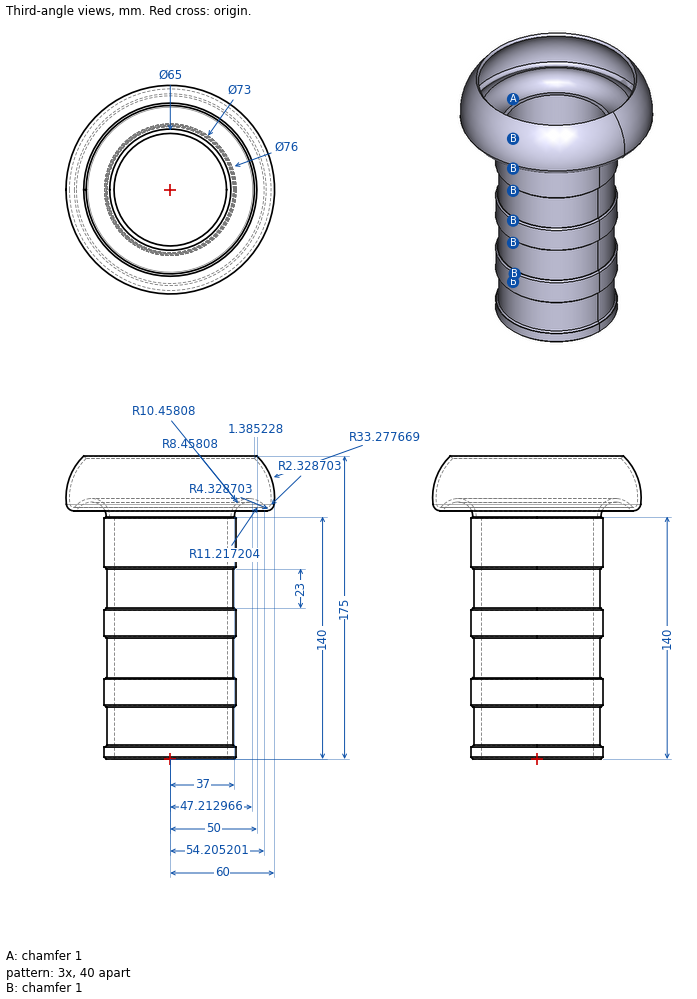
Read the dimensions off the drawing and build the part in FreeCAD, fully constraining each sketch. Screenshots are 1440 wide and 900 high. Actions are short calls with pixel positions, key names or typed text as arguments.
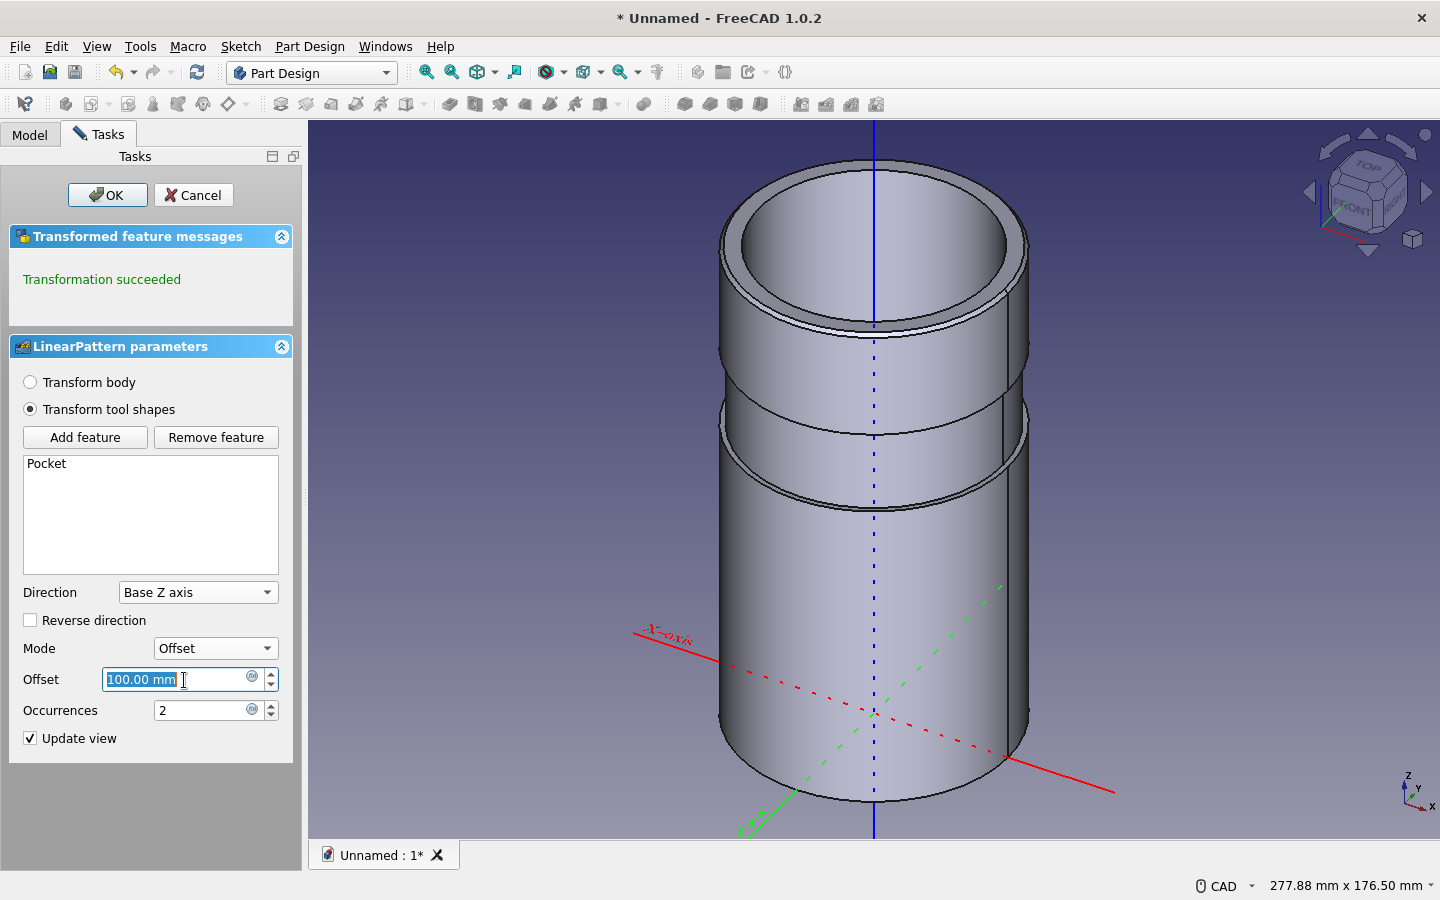
text(40)
key(Tab)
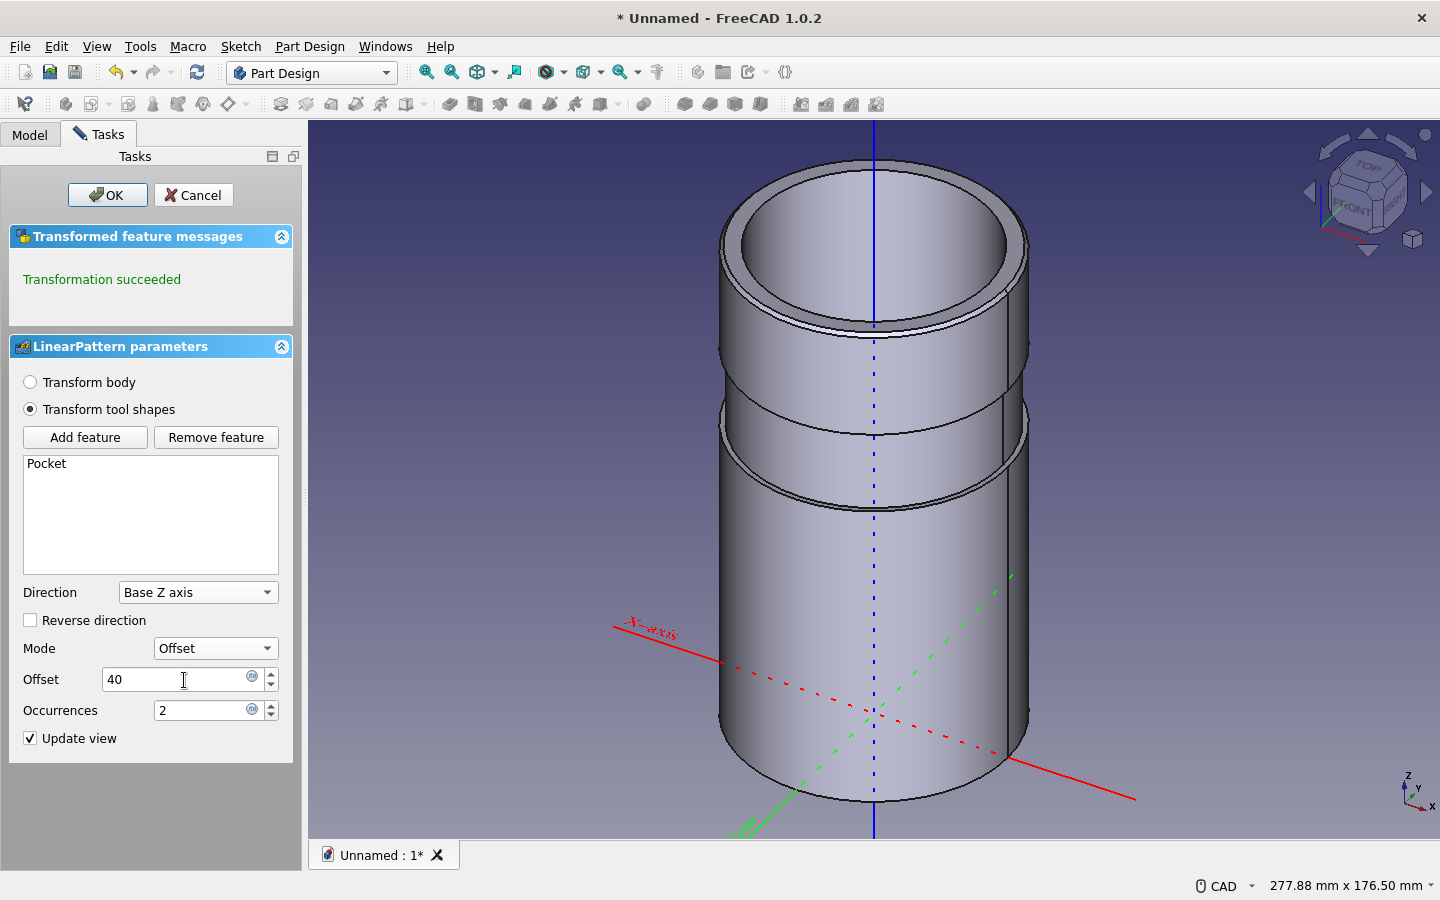
triple_click(210, 710)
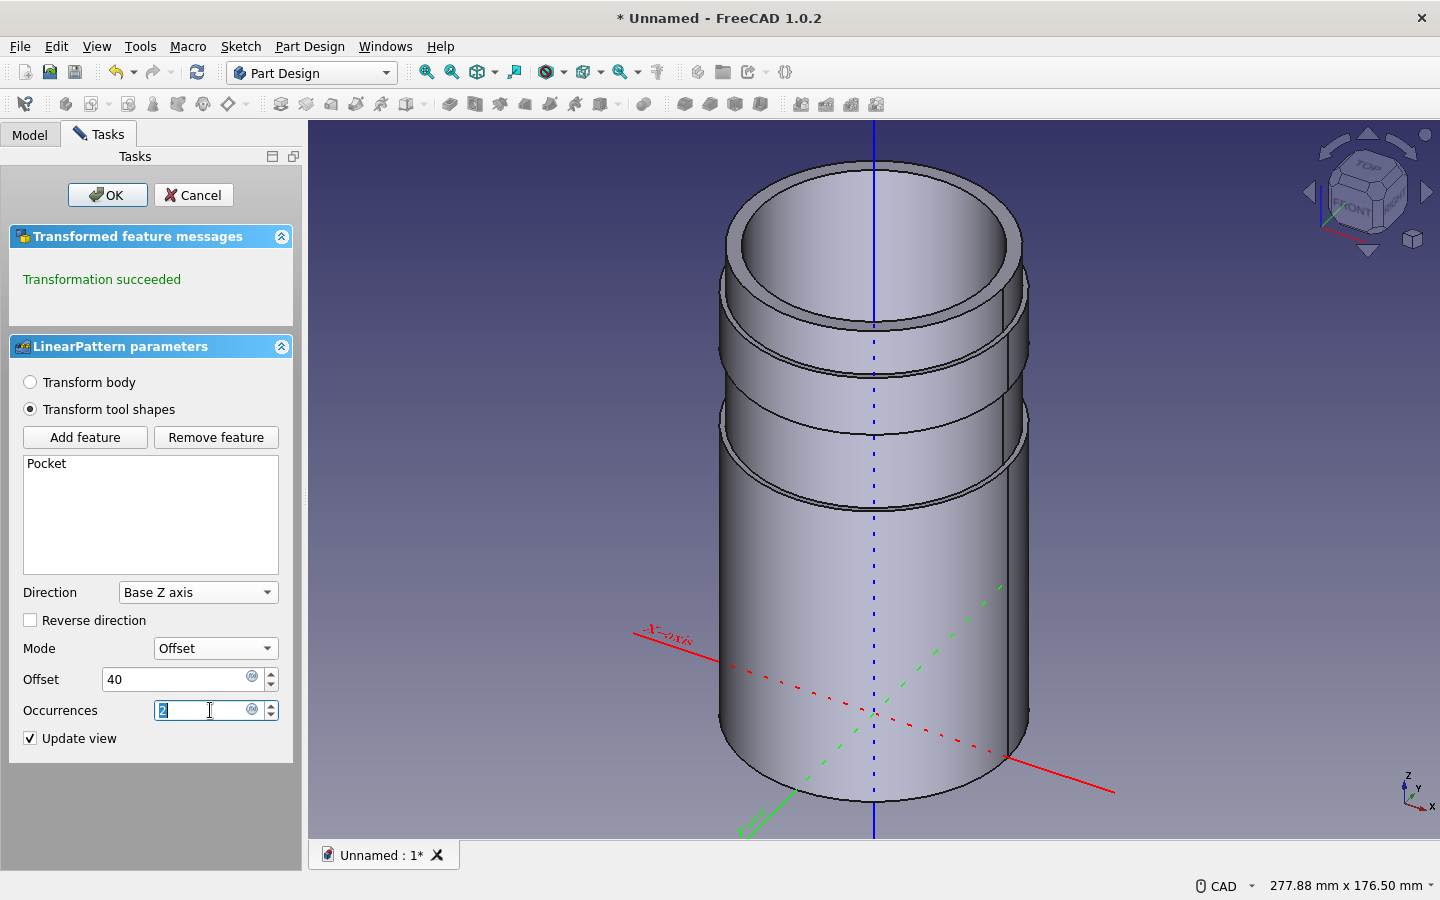
text(3)
key(Tab)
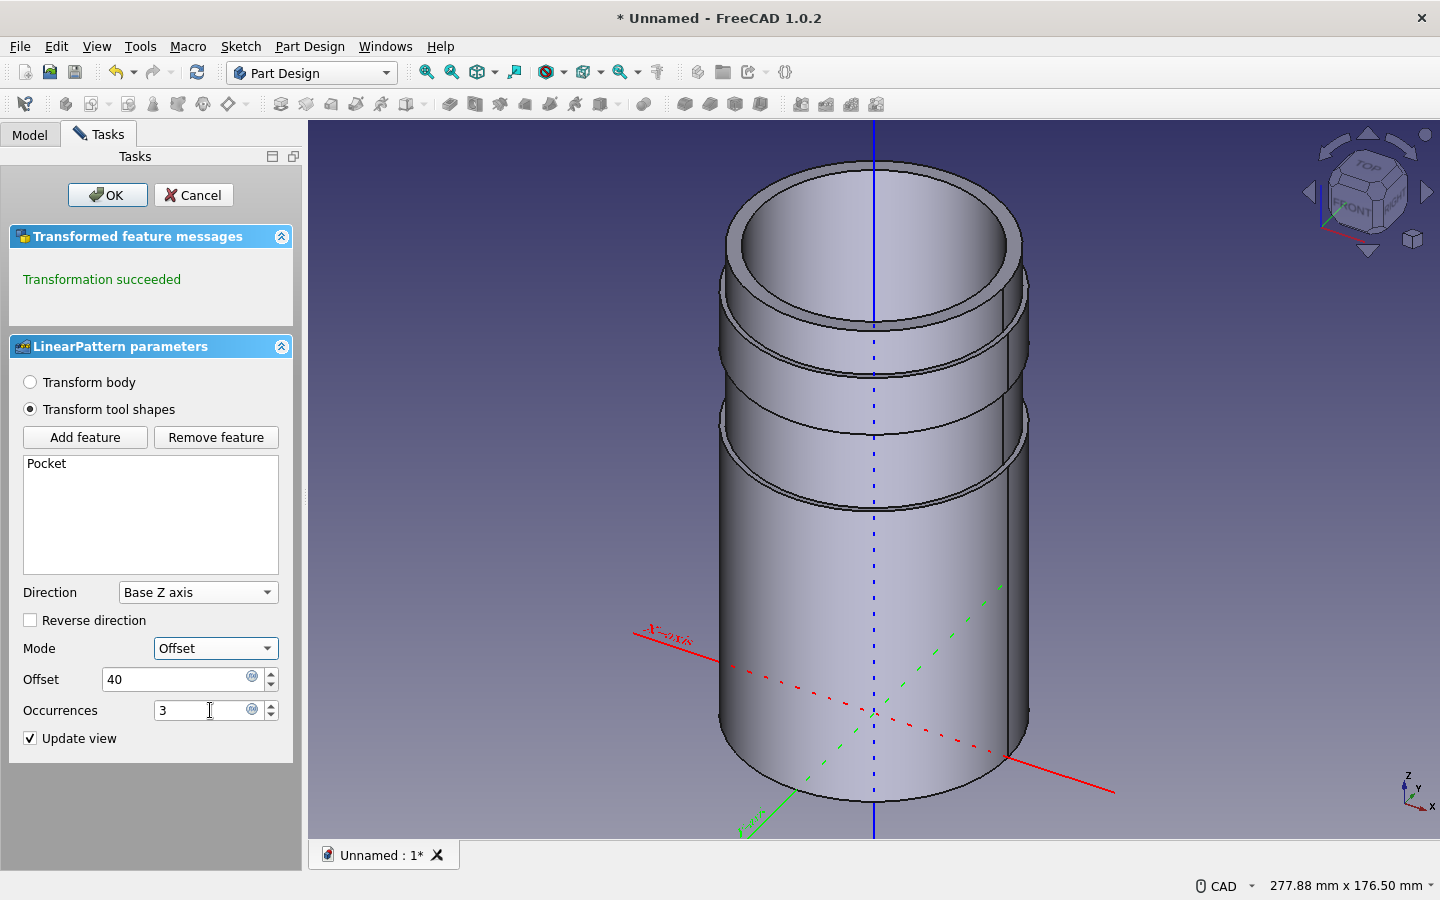
click(31, 620)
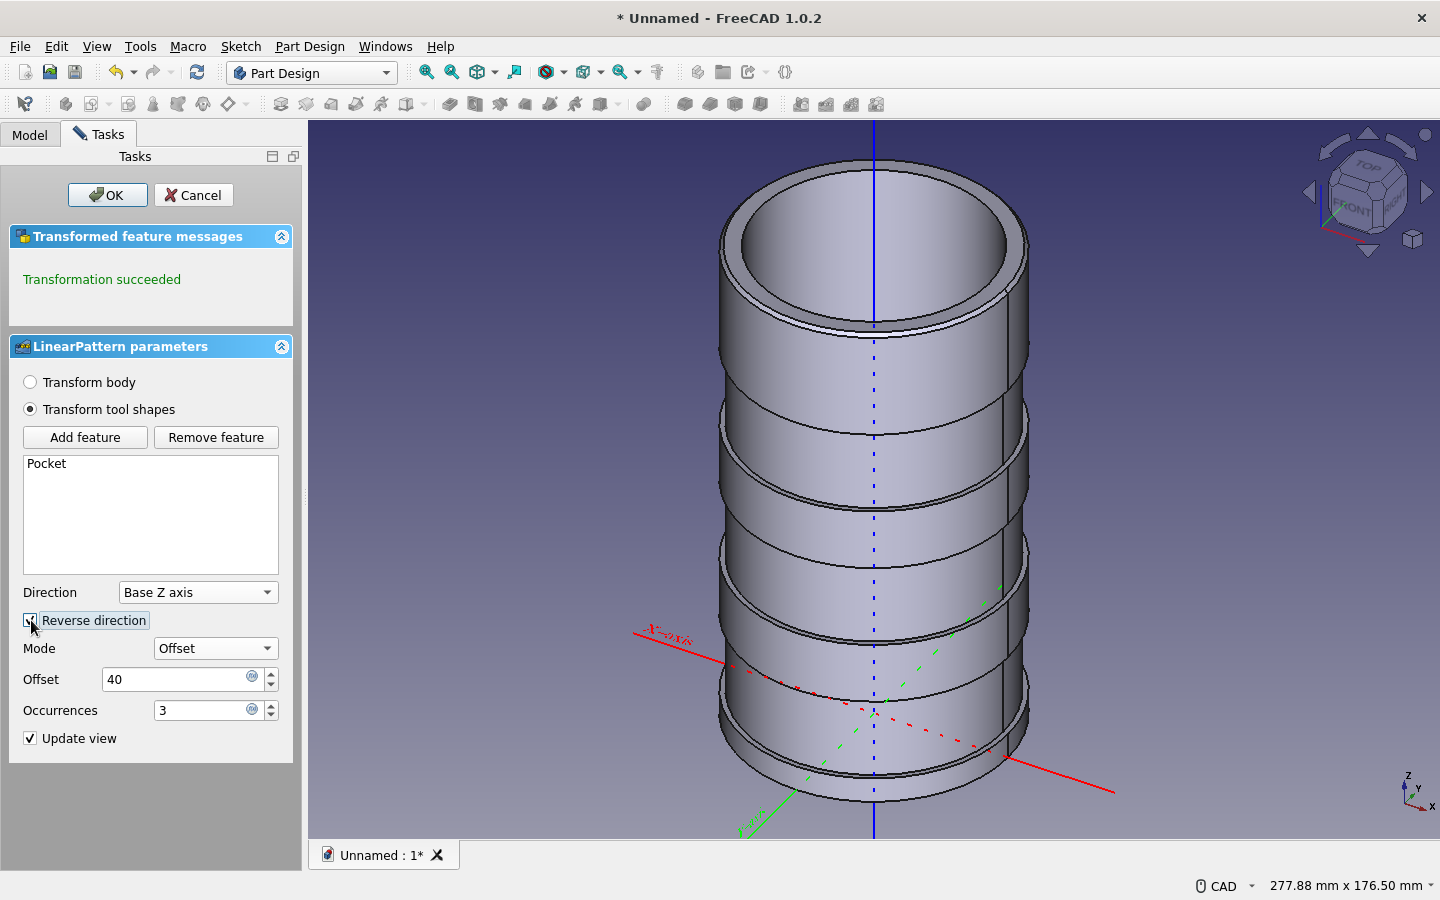
click(108, 195)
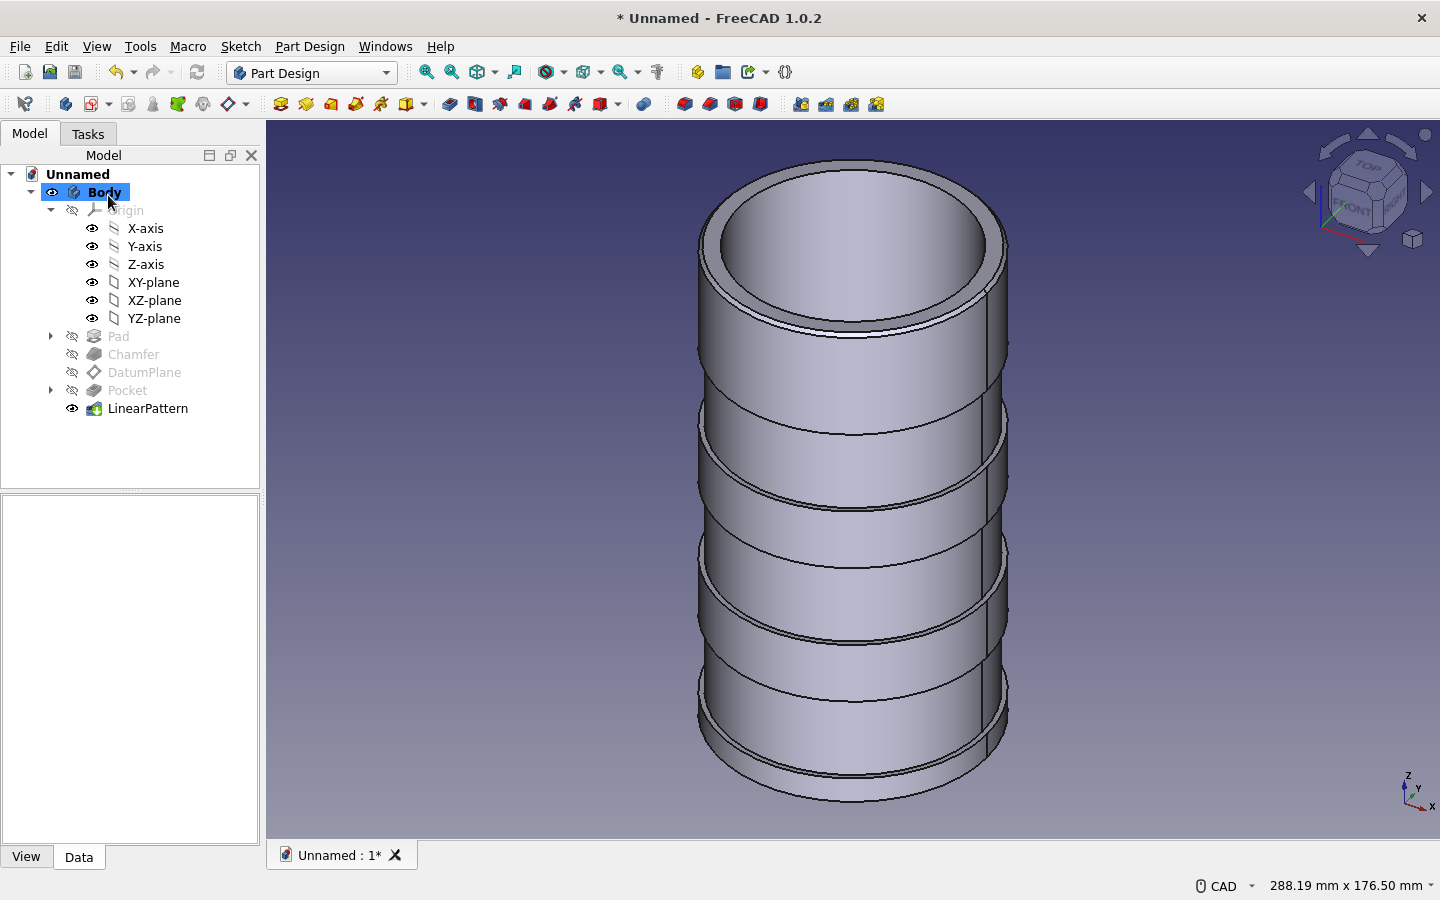
click(699, 431)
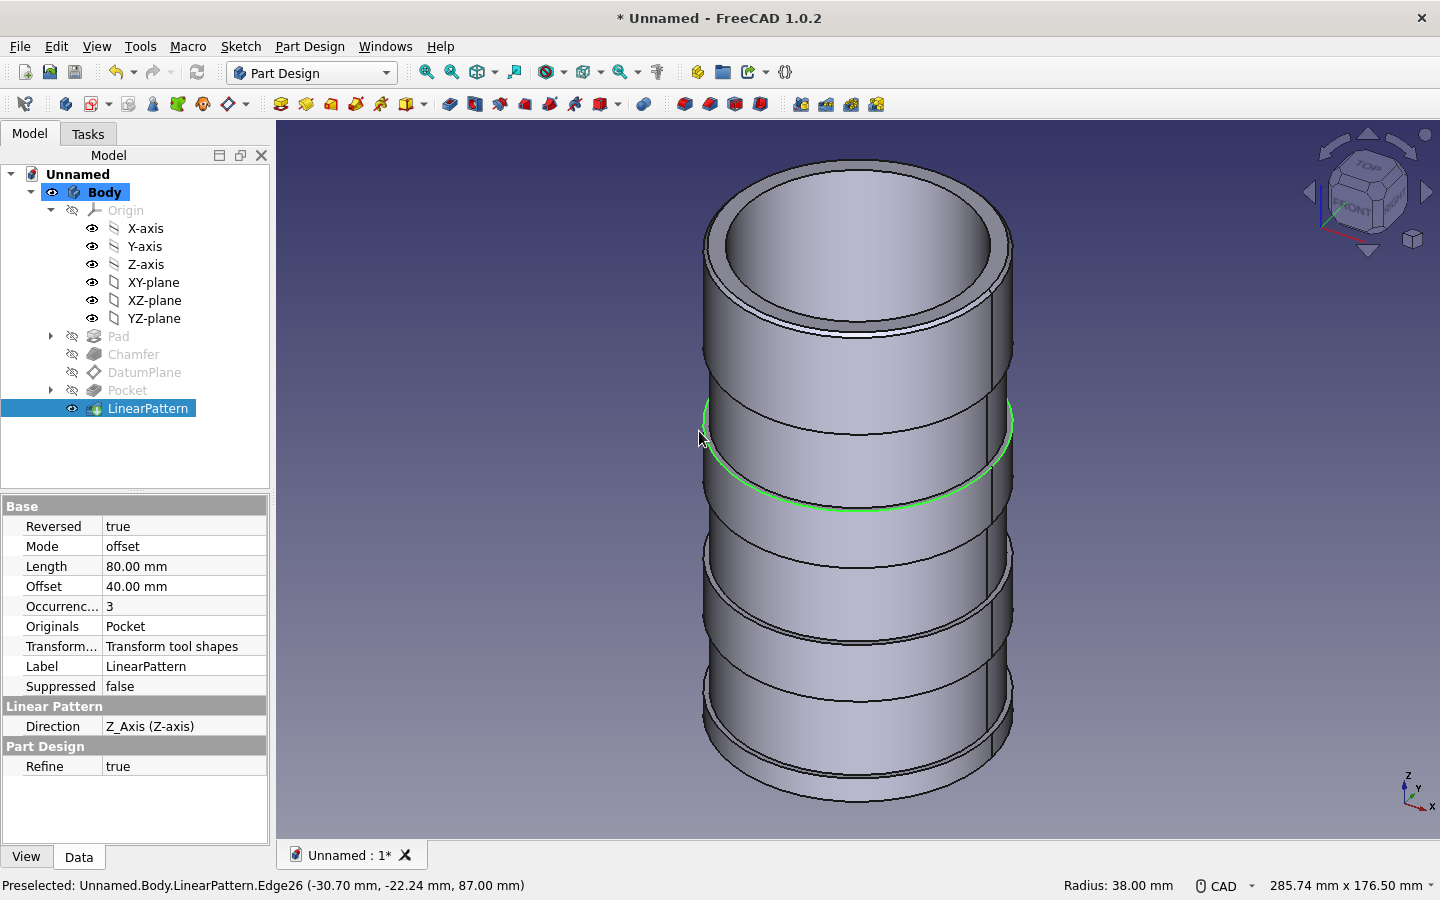
click(704, 565, ctrl)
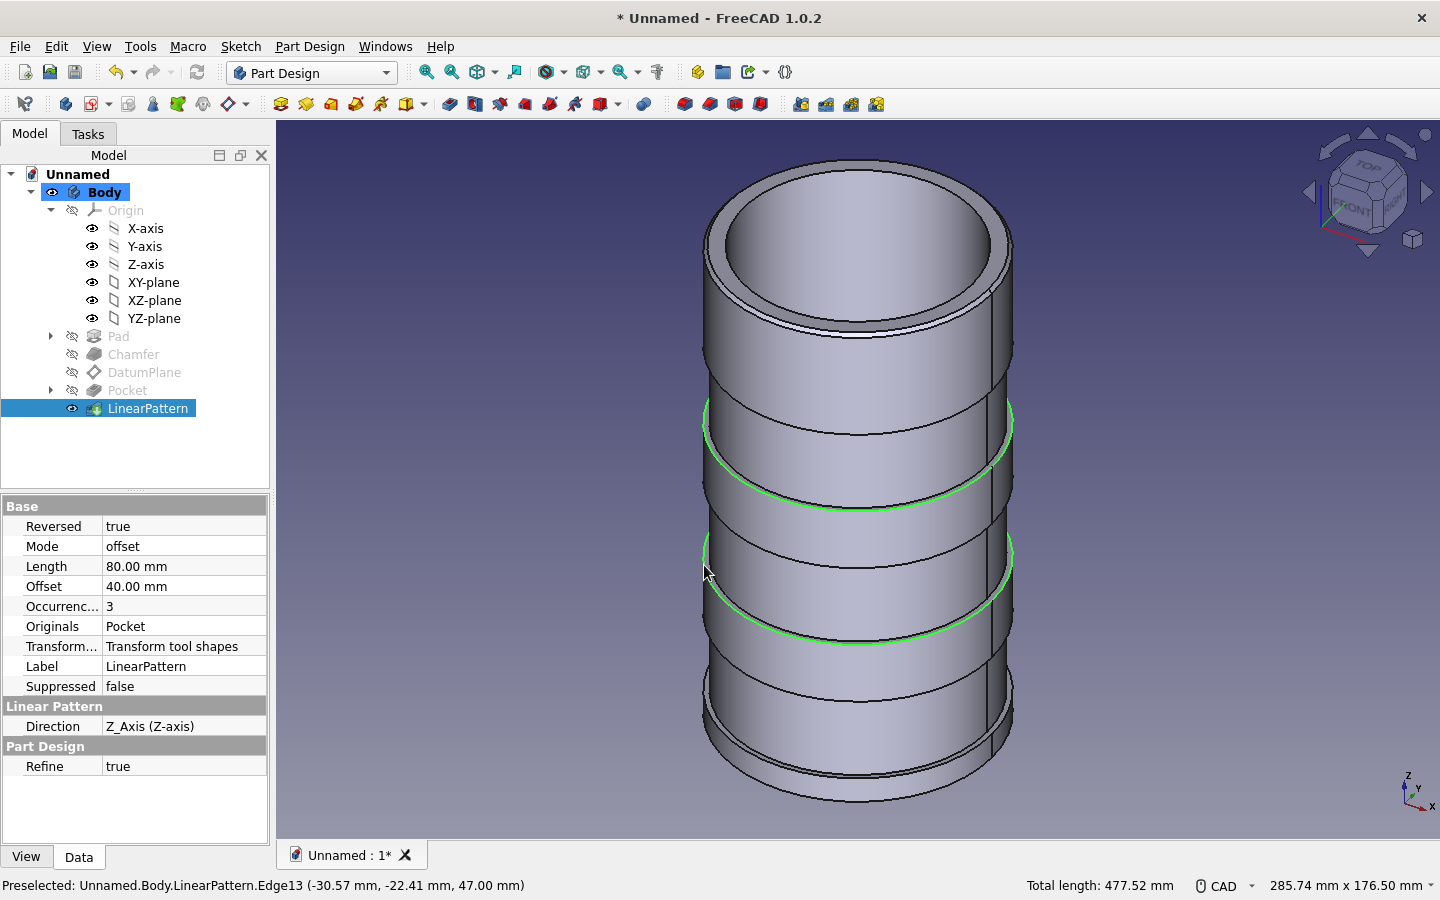
key(0)